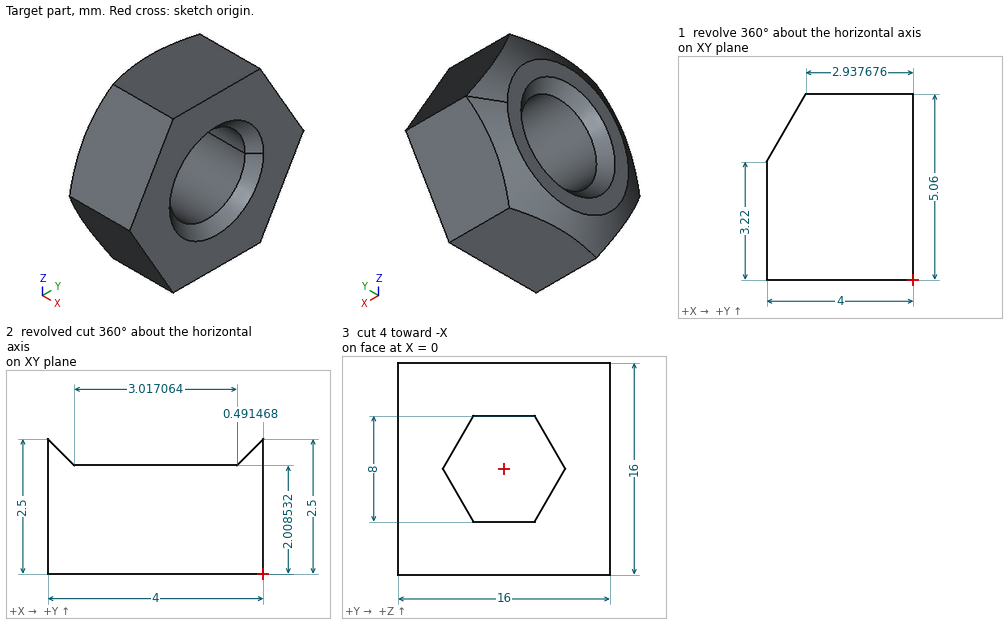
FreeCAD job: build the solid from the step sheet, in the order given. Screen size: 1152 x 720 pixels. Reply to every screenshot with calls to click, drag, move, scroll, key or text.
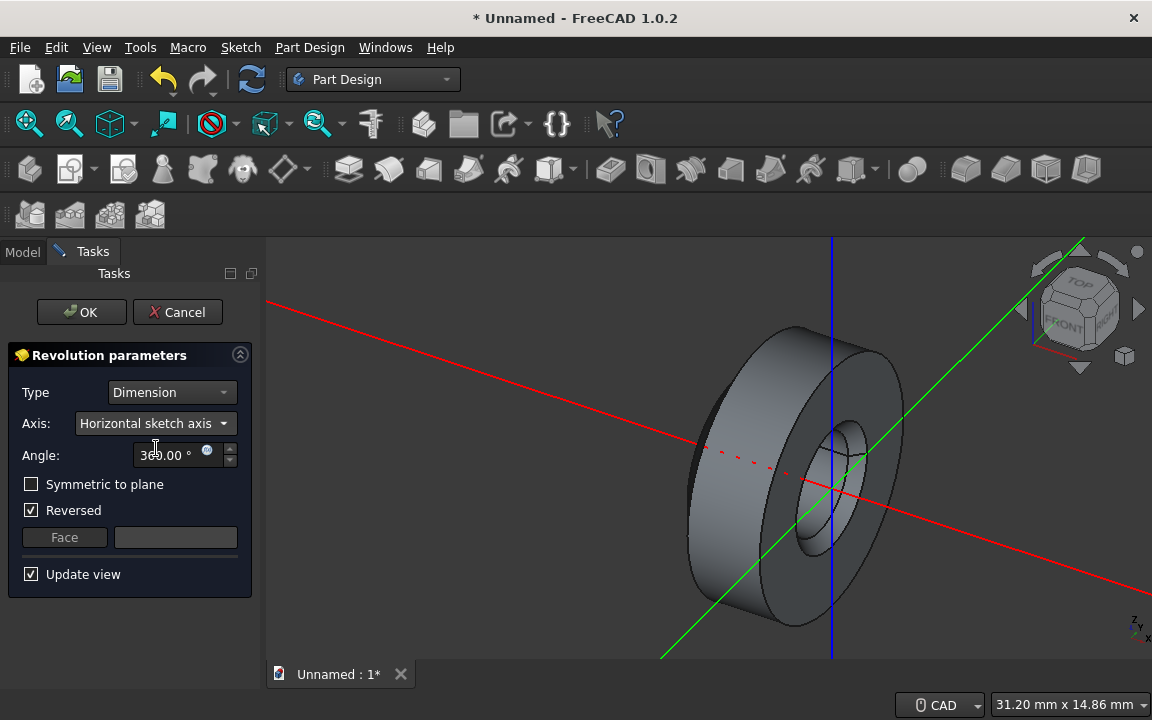
click(82, 312)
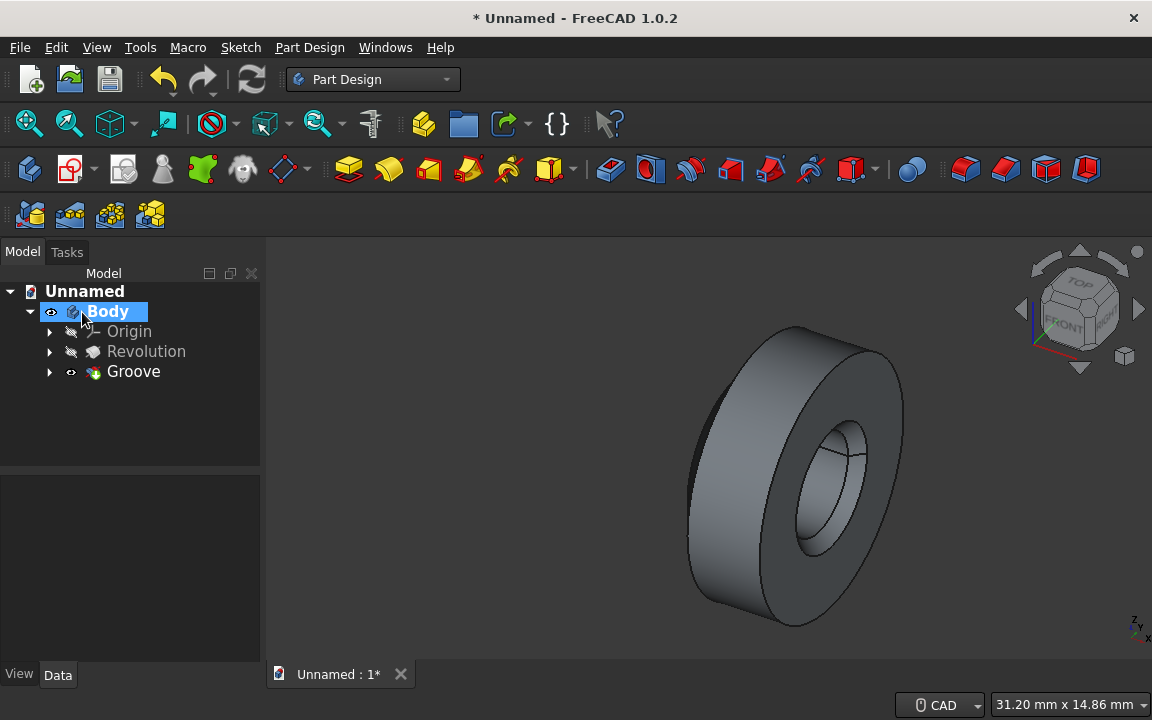
key(v)
key(f)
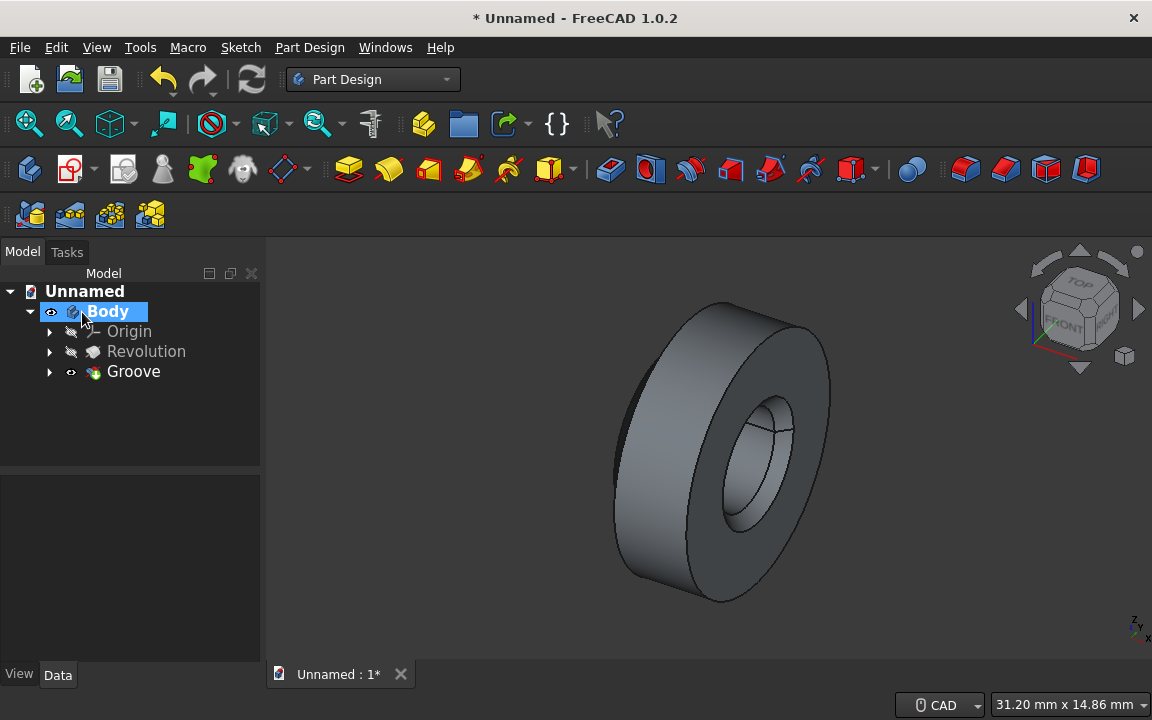
click(799, 490)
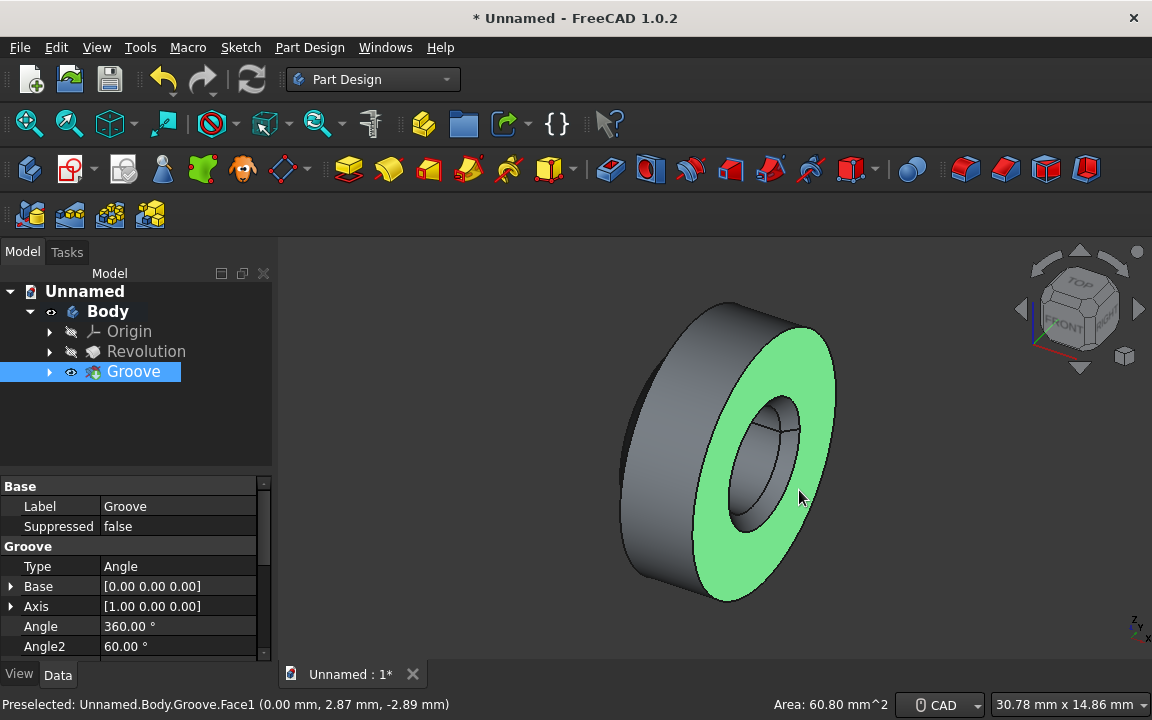
click(70, 170)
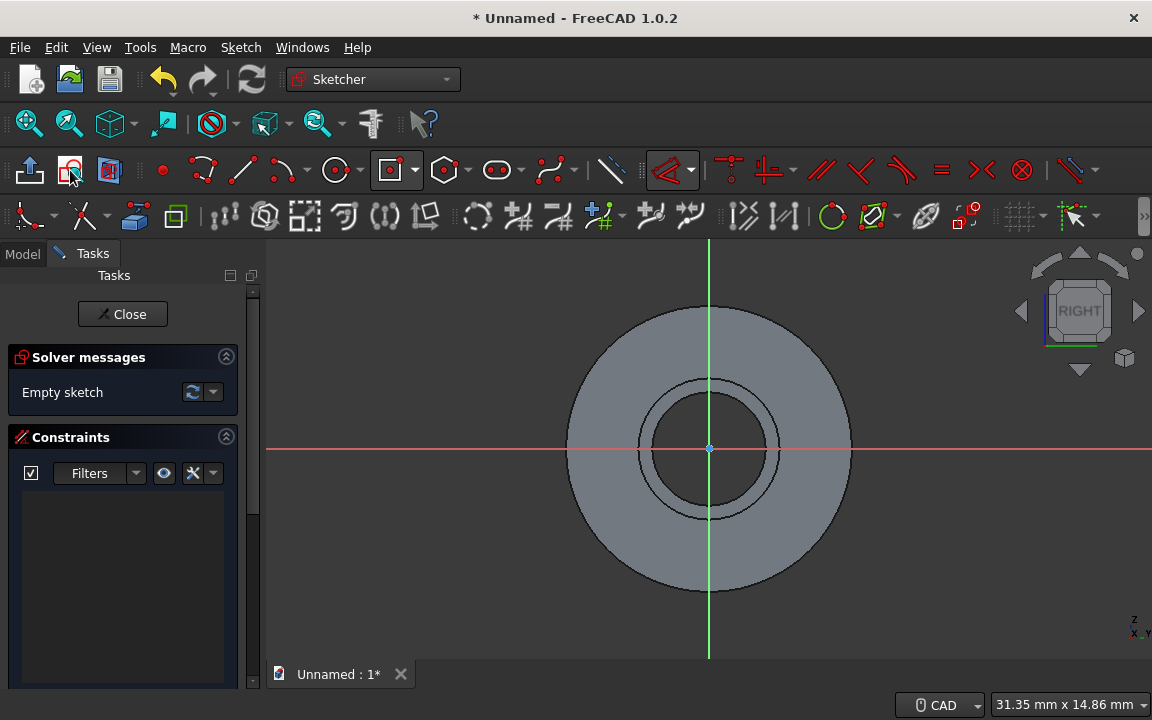
scroll(557, 449, down, 3)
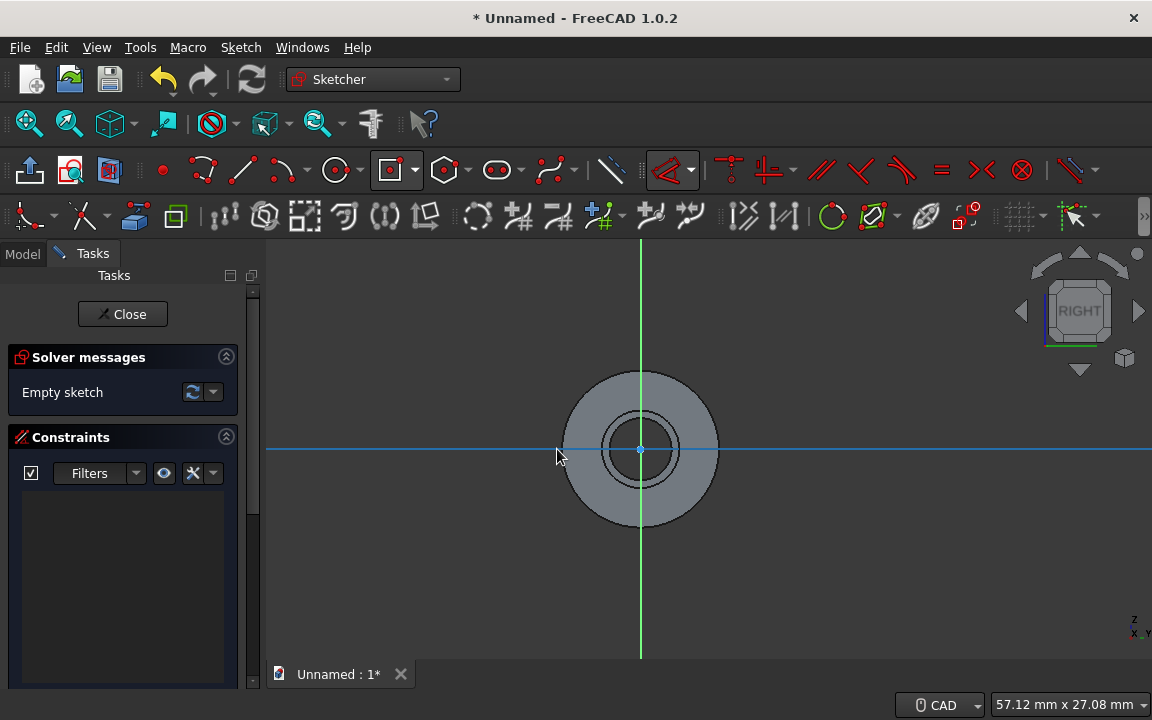
key(g)
key(v)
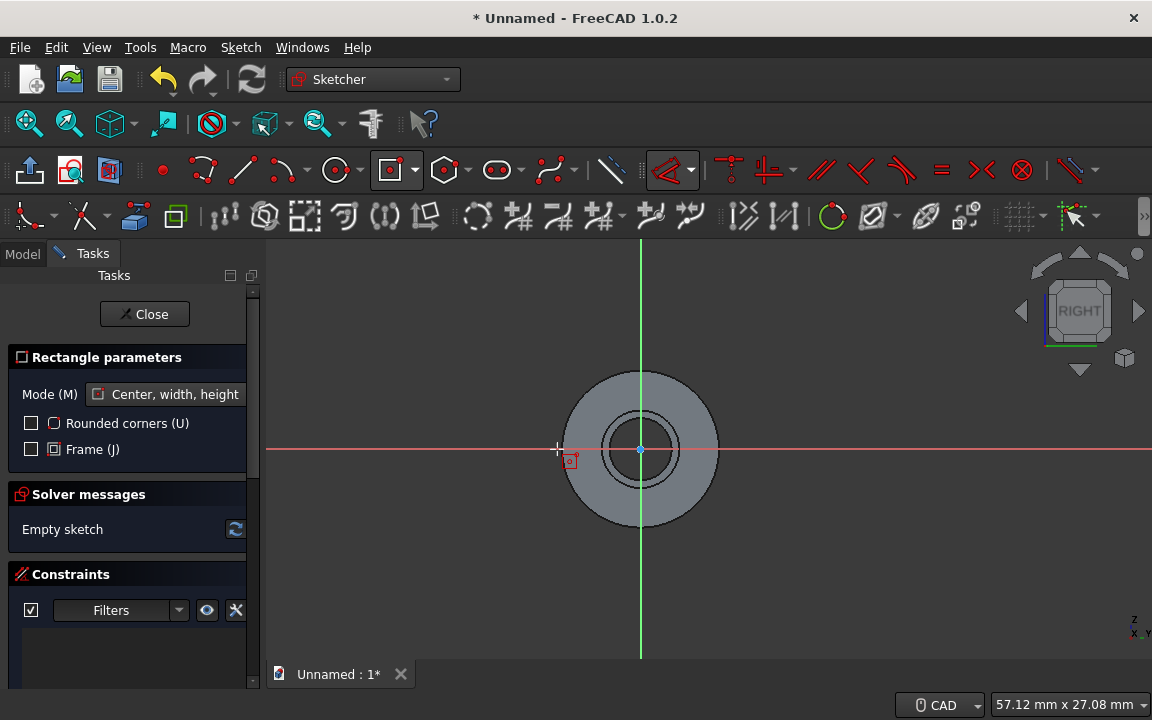
click(641, 449)
click(765, 325)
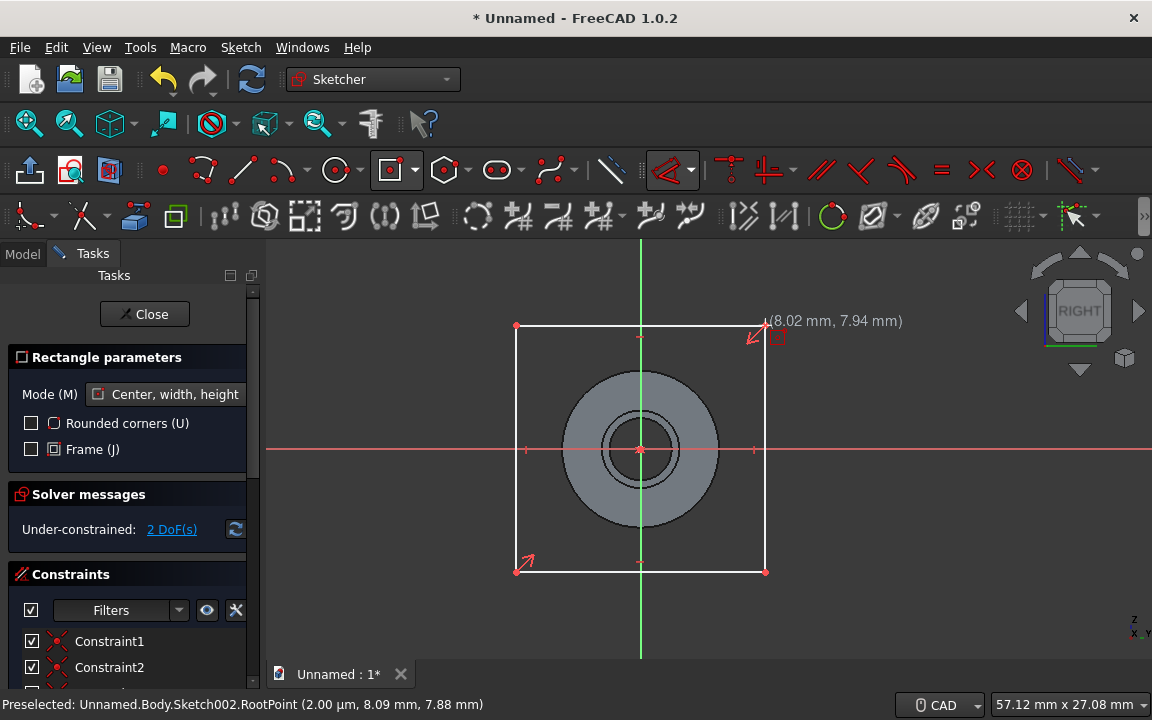
click(444, 170)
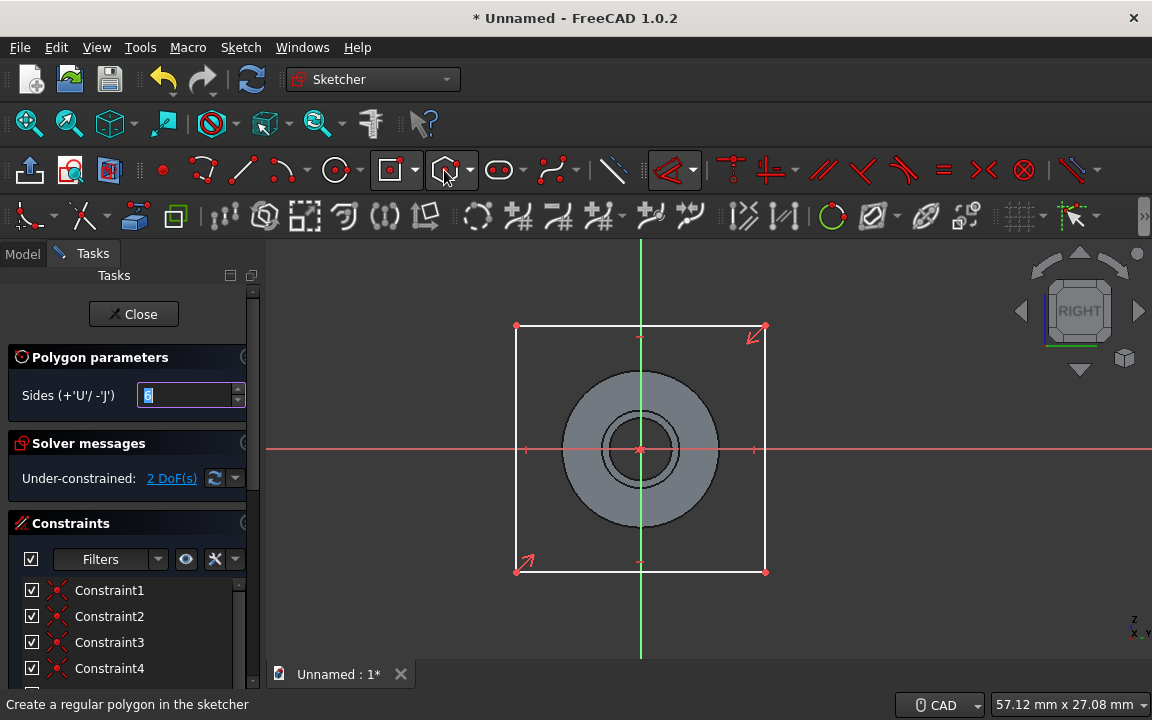
click(641, 449)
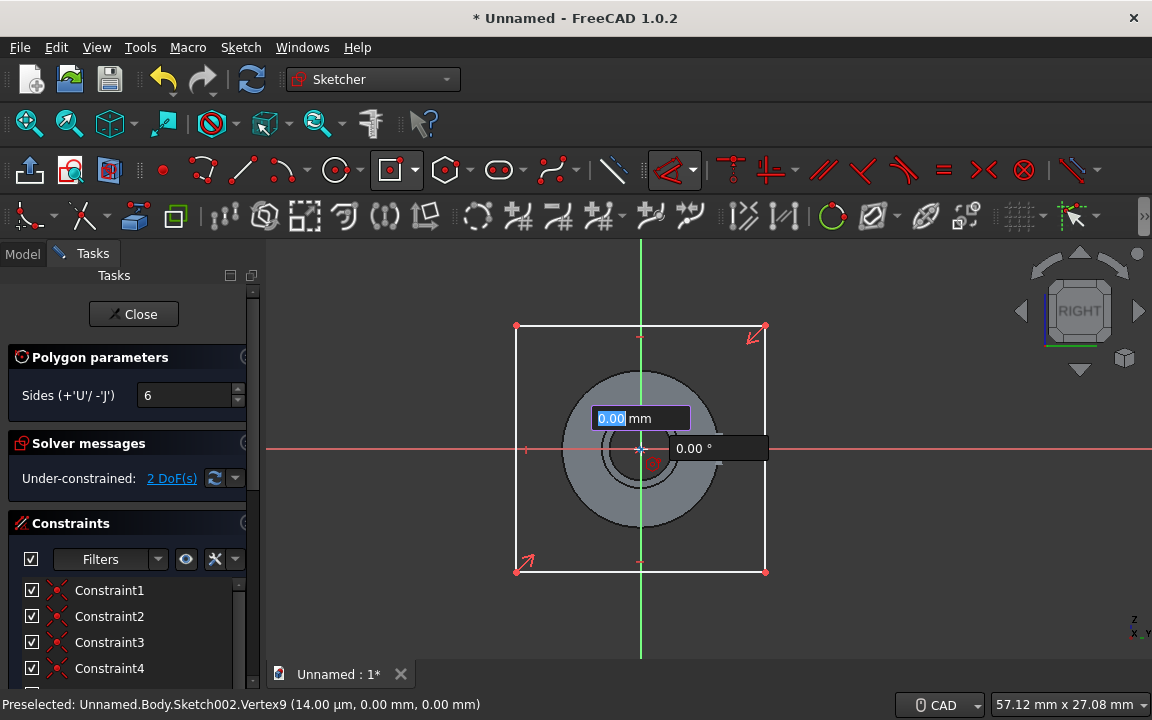
click(712, 449)
right_click(712, 449)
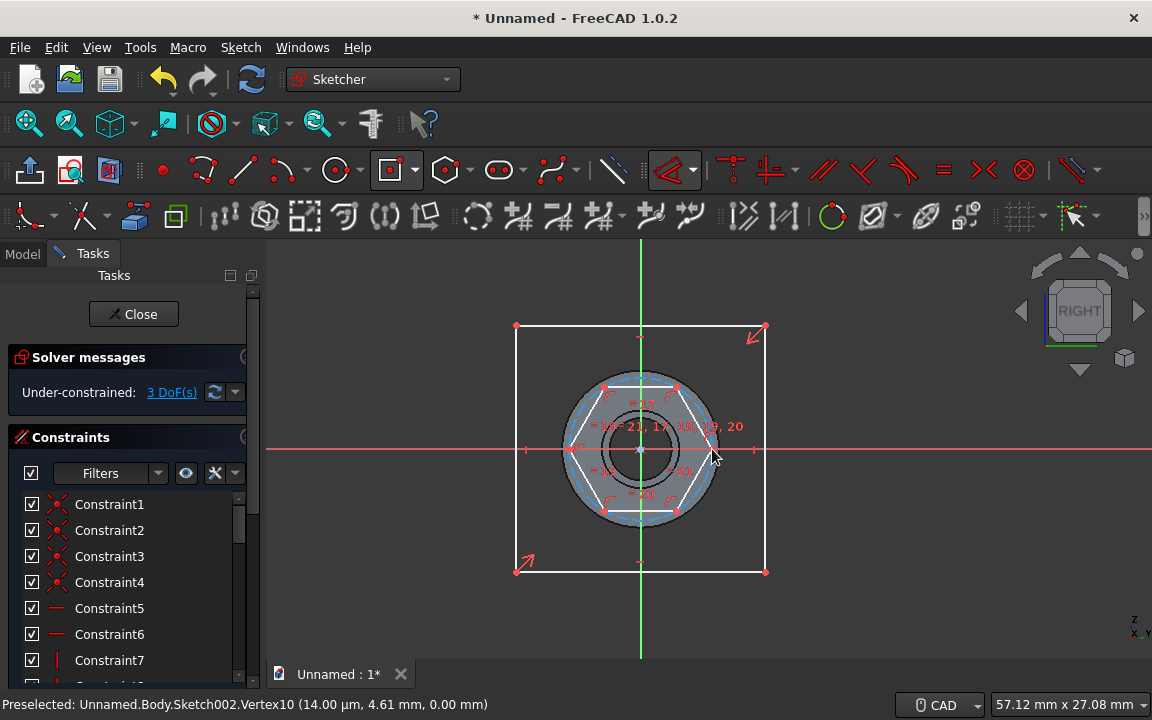
click(605, 511)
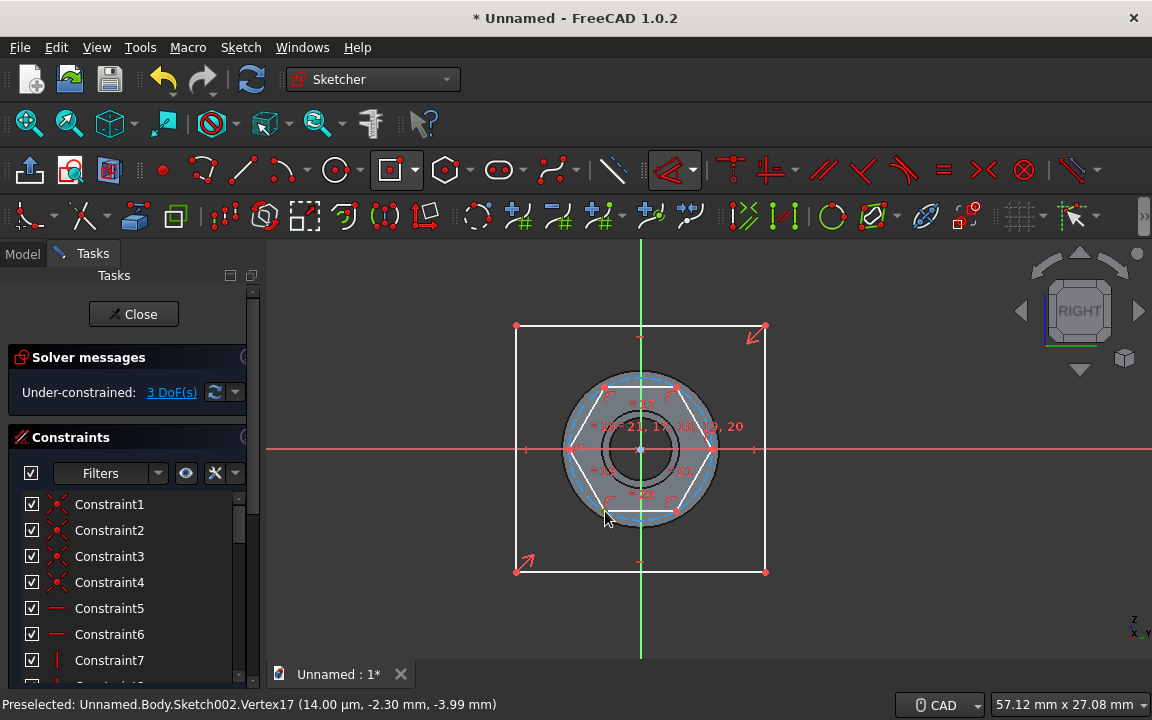
click(676, 387)